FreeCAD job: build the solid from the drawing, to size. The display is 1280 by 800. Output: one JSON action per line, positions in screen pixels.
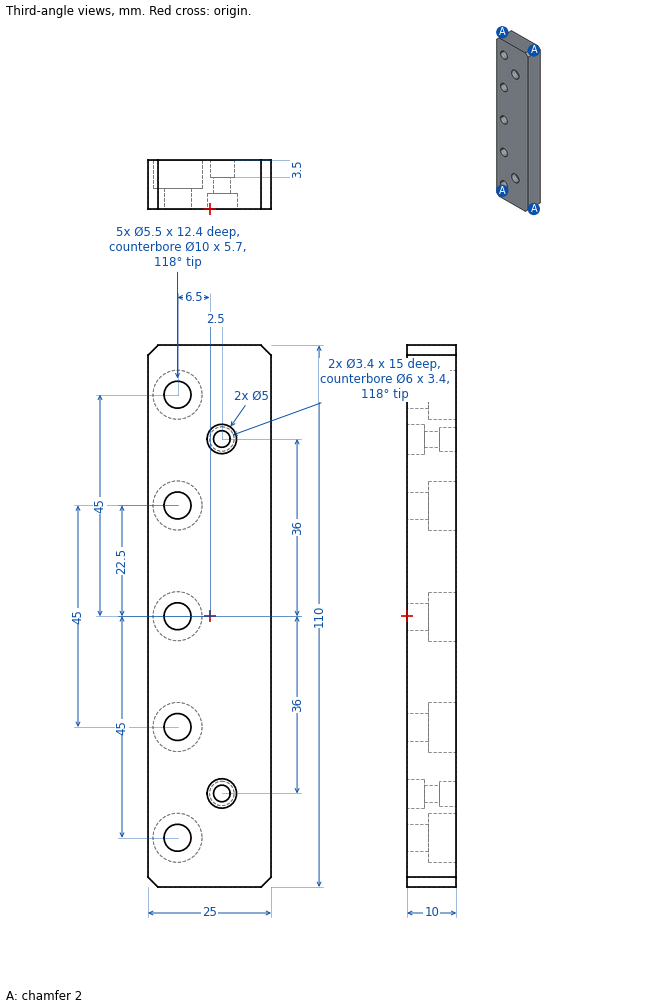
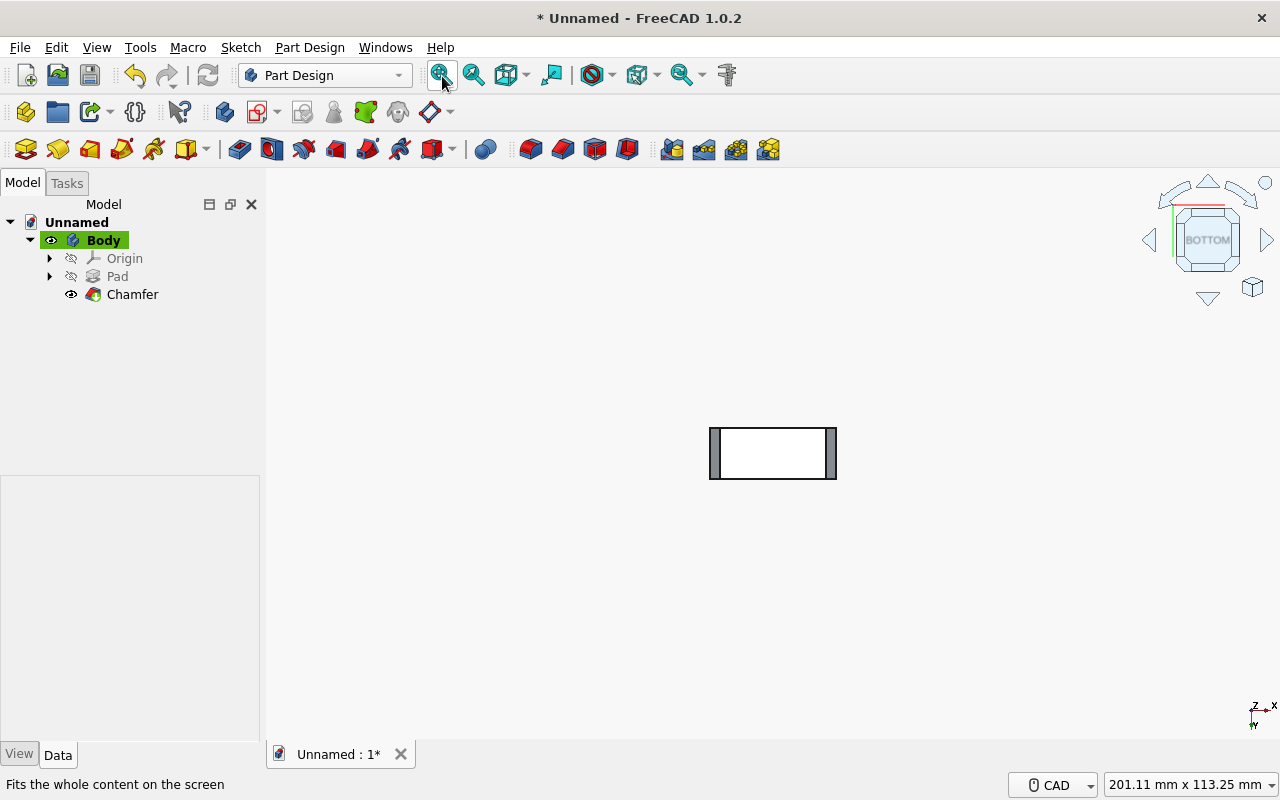
{"action": "key", "text": "4"}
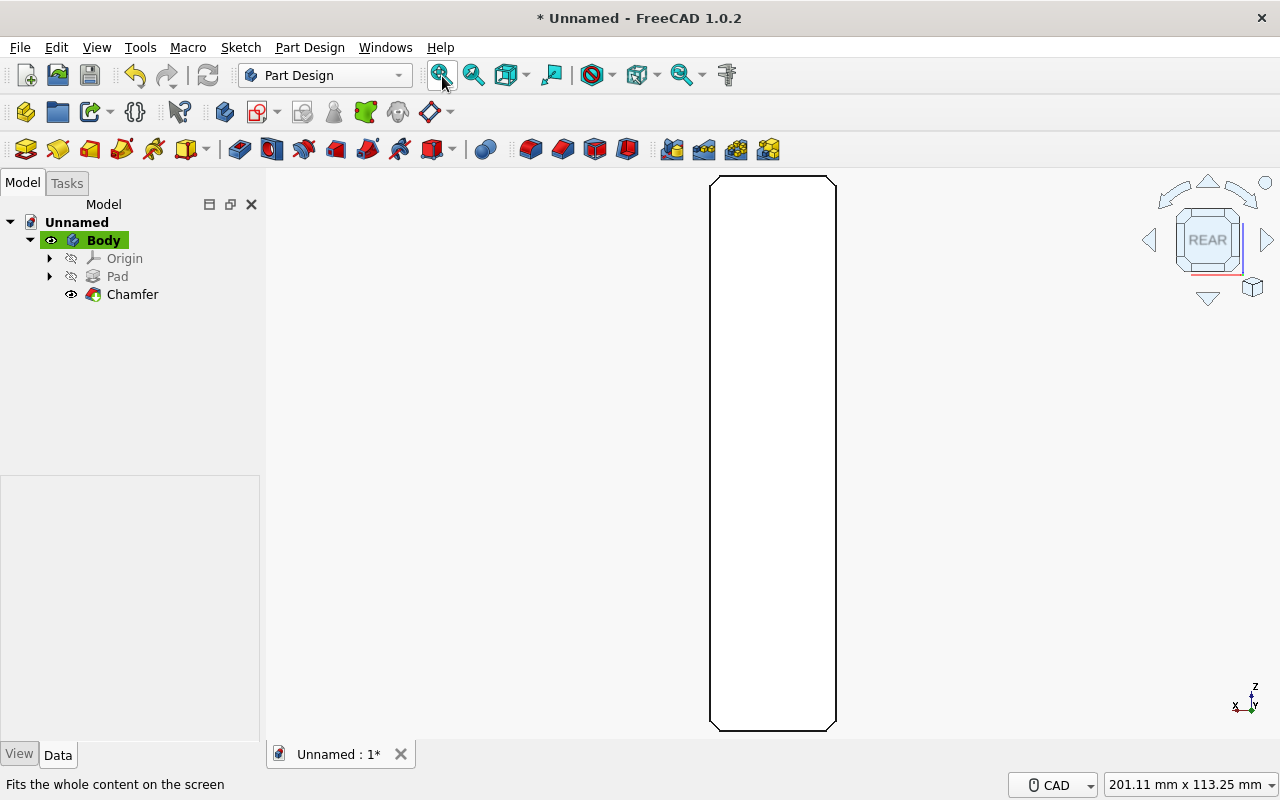
{"action": "left_click", "coordinate": [773, 294]}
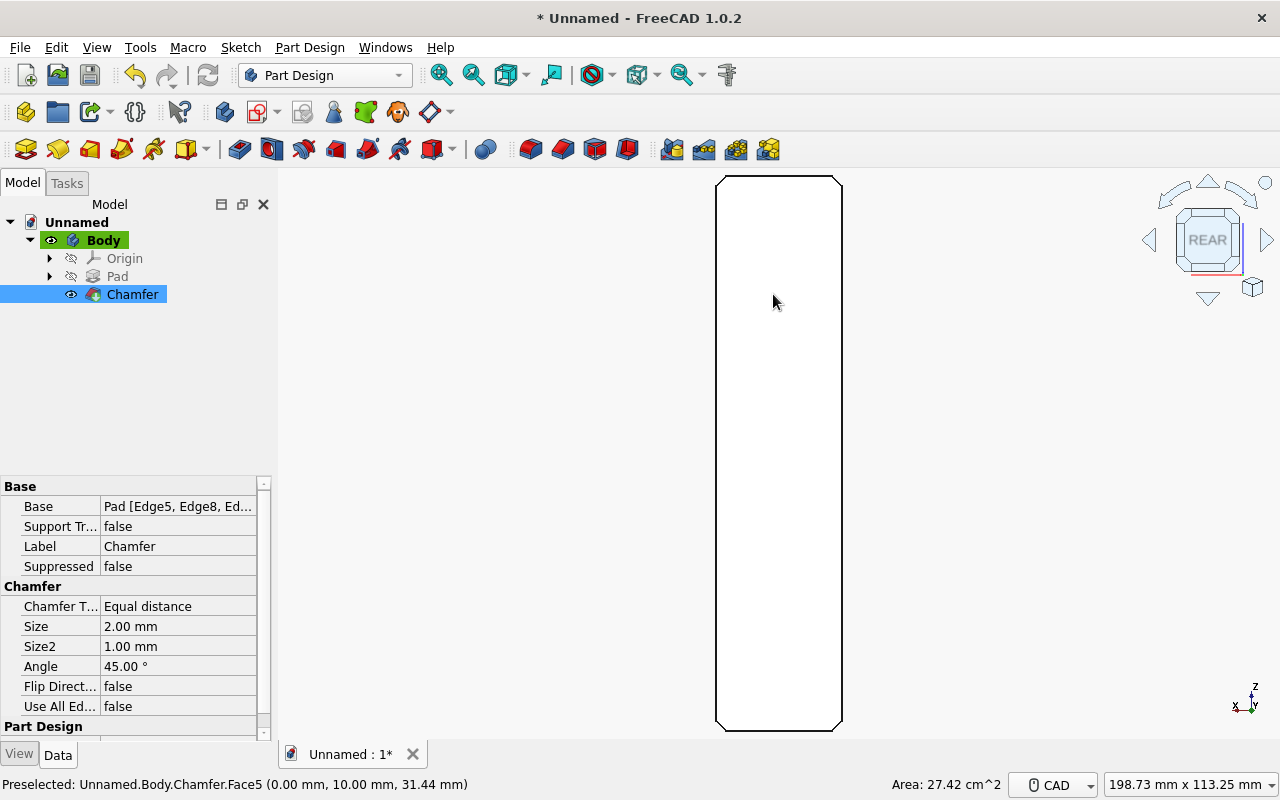
{"action": "left_click", "coordinate": [258, 112]}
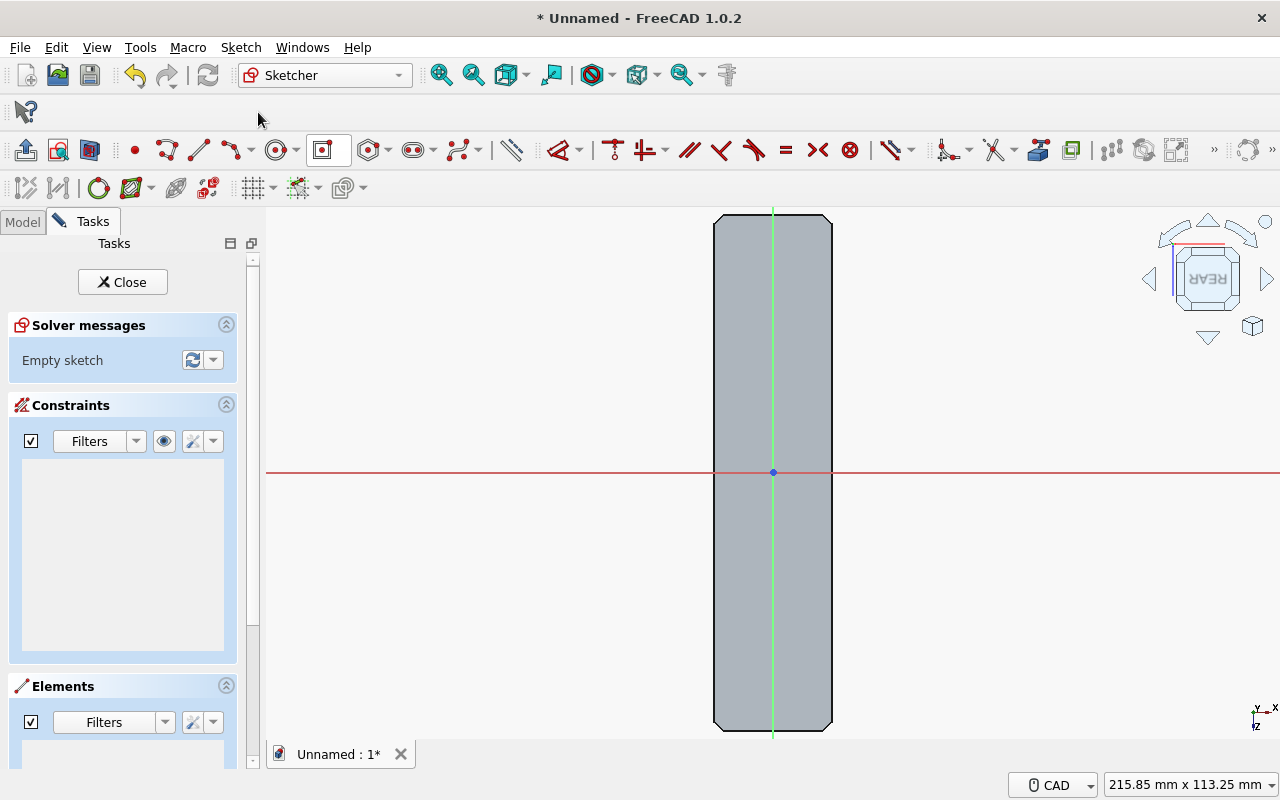
{"action": "scroll", "coordinate": [493, 473], "scroll_direction": "down", "scroll_amount": 1}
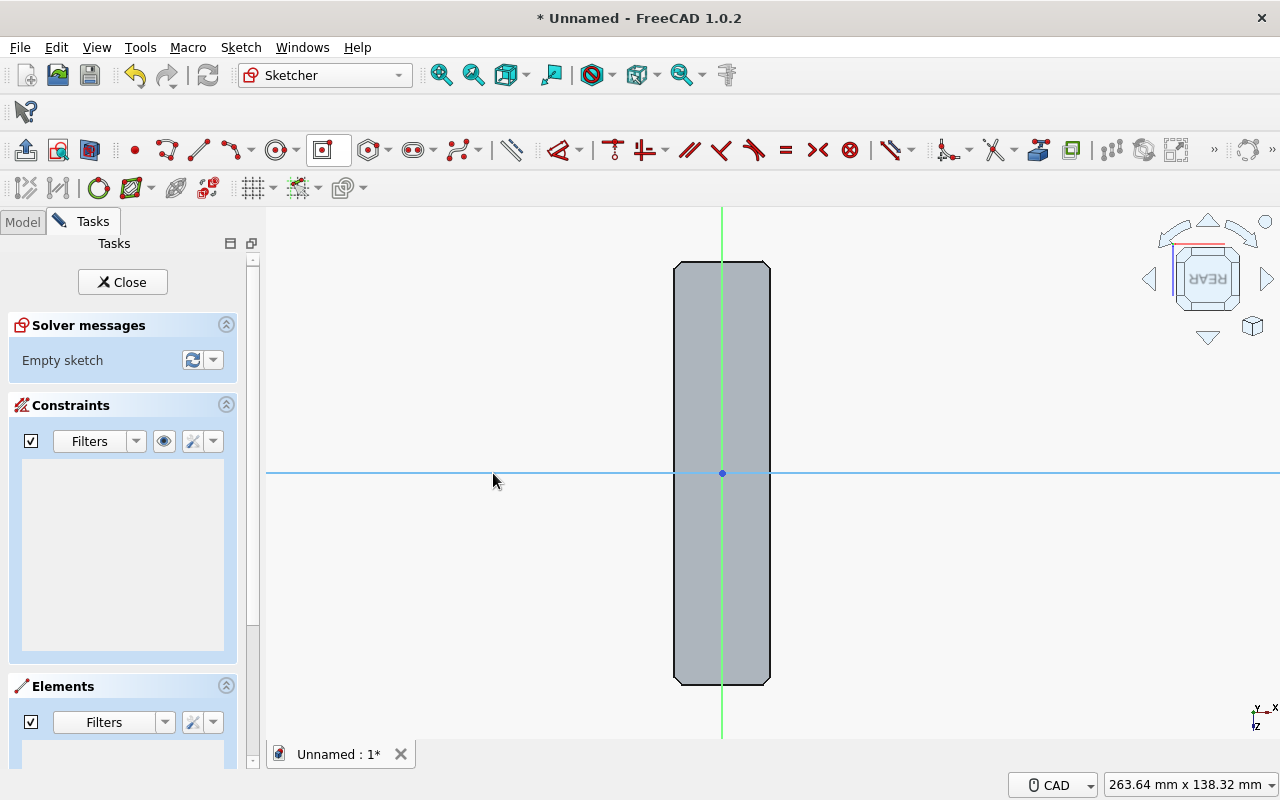
{"action": "left_click", "coordinate": [276, 150]}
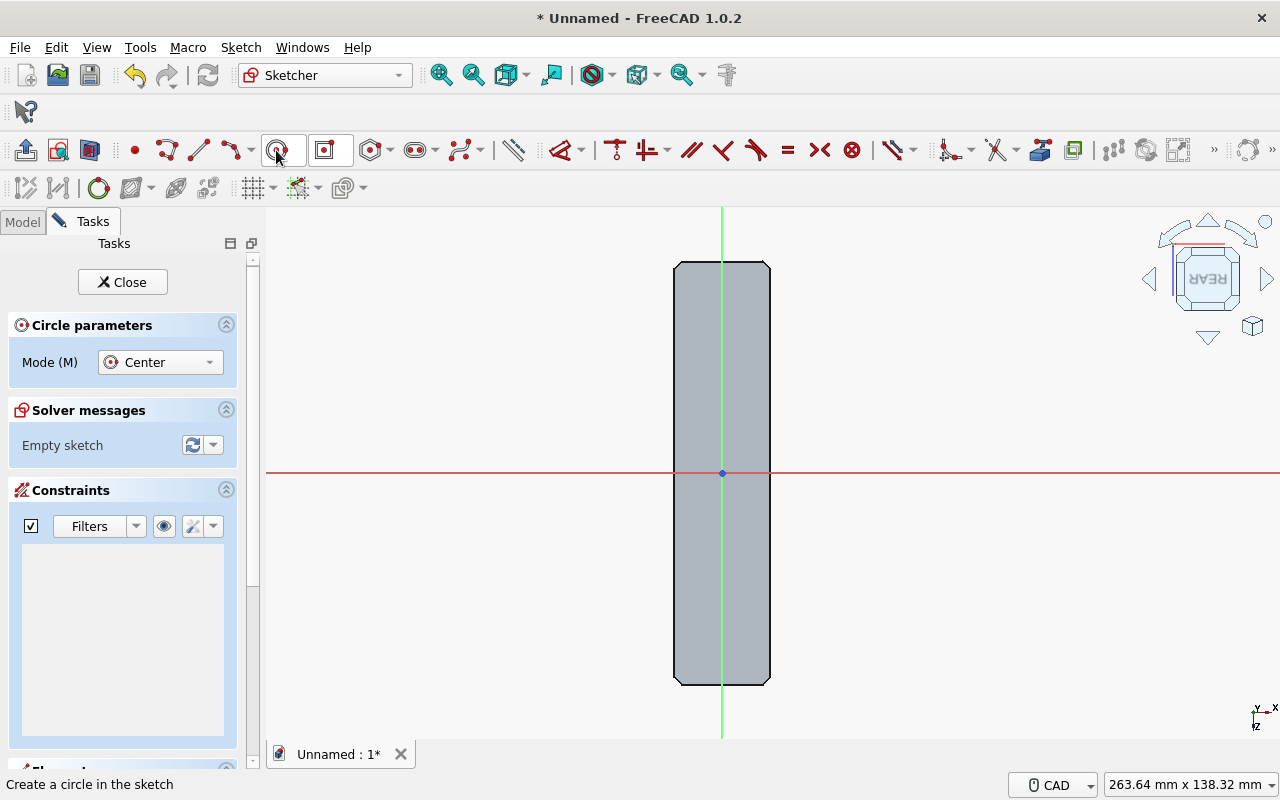
{"action": "scroll", "coordinate": [697, 646], "scroll_direction": "up", "scroll_amount": 4}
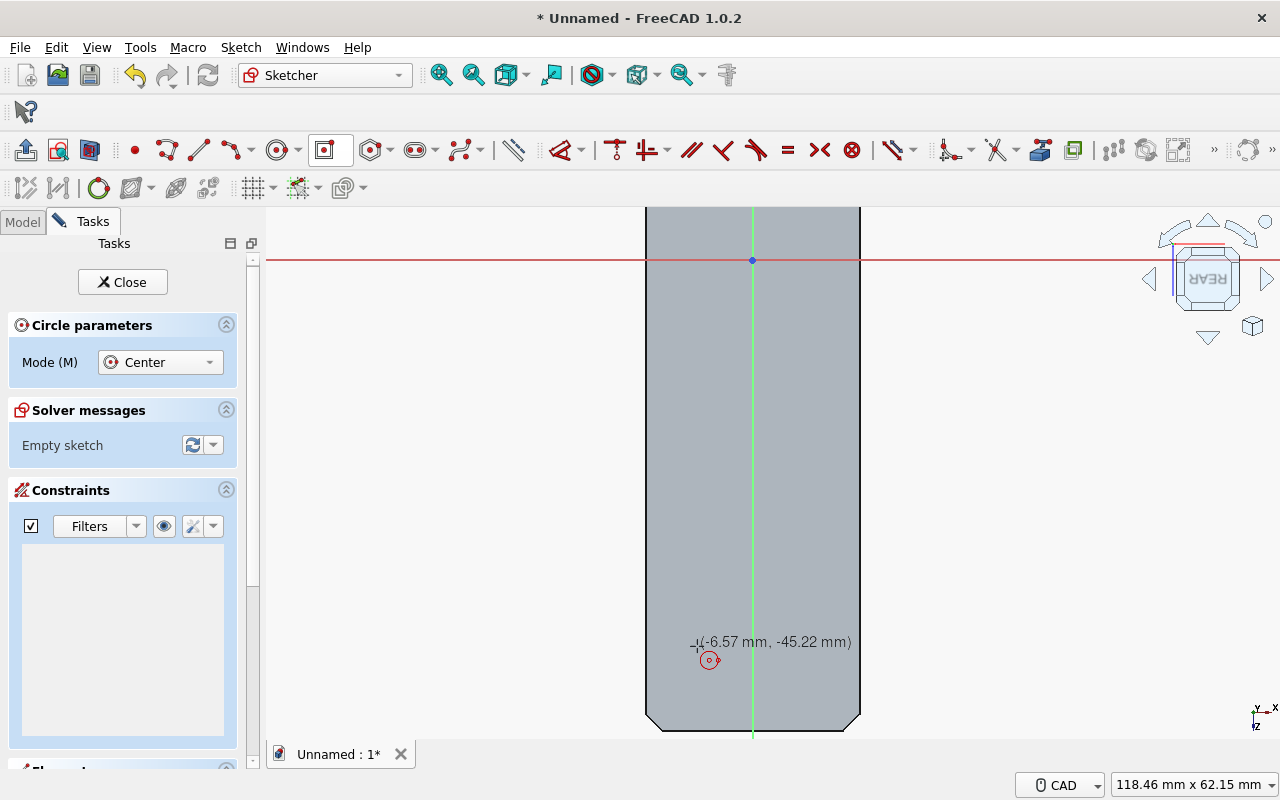
{"action": "left_click", "coordinate": [697, 645]}
{"action": "mouse_move", "coordinate": [714, 629]}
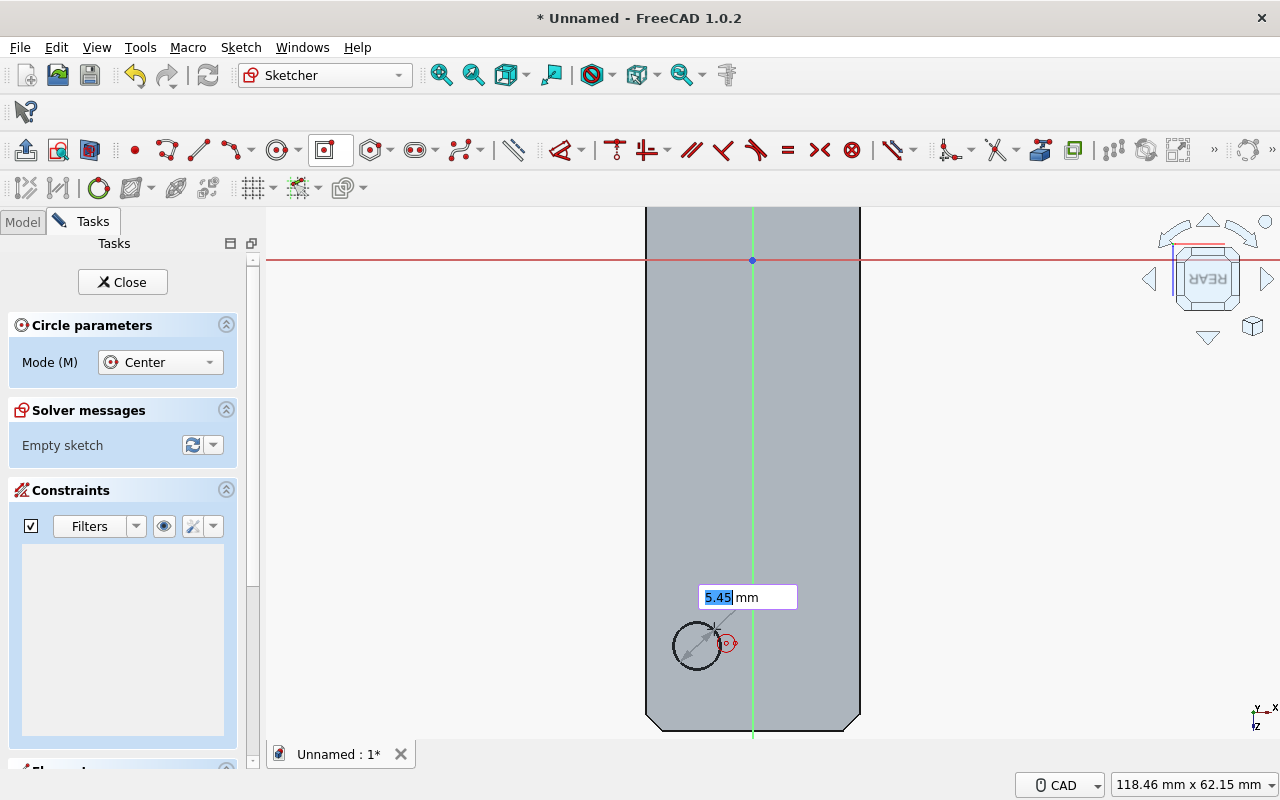
{"action": "type", "text": "5.5"}
{"action": "key", "text": "Return"}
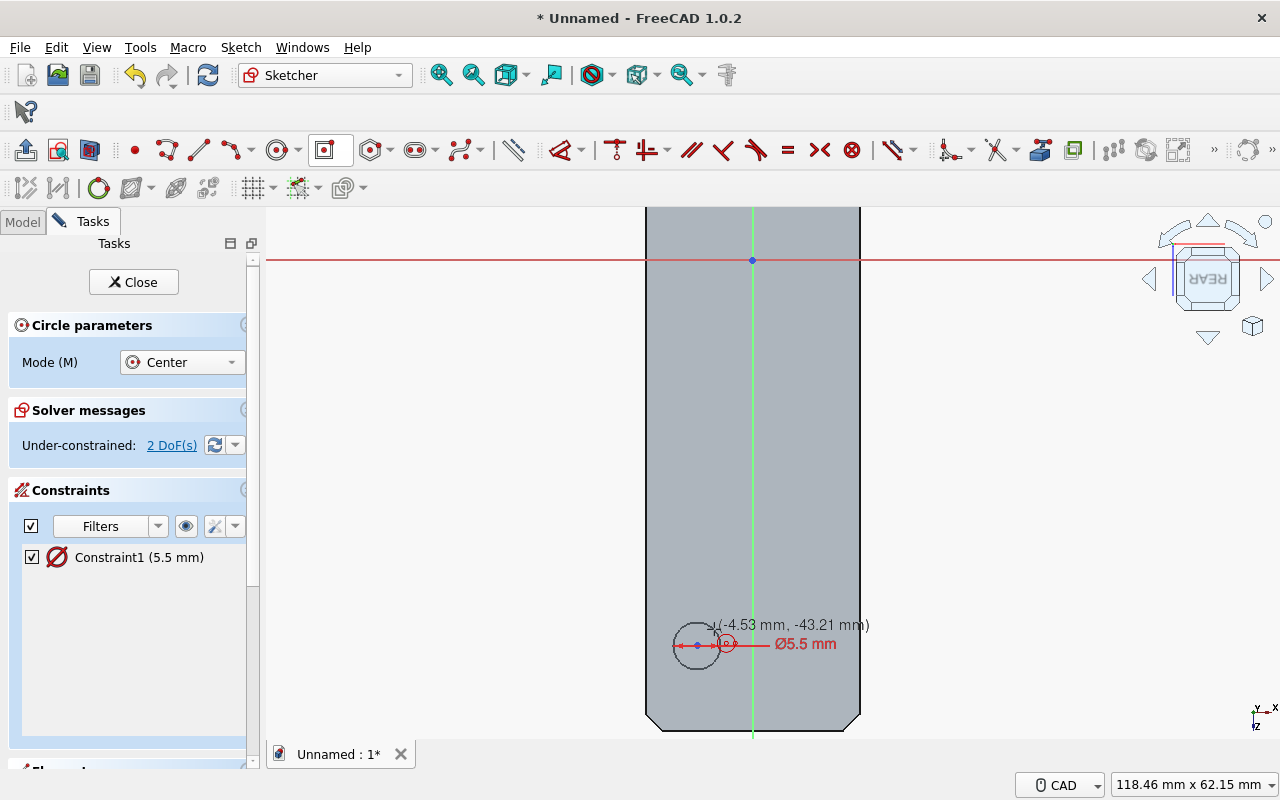
{"action": "left_click", "coordinate": [697, 260]}
{"action": "mouse_move", "coordinate": [714, 244]}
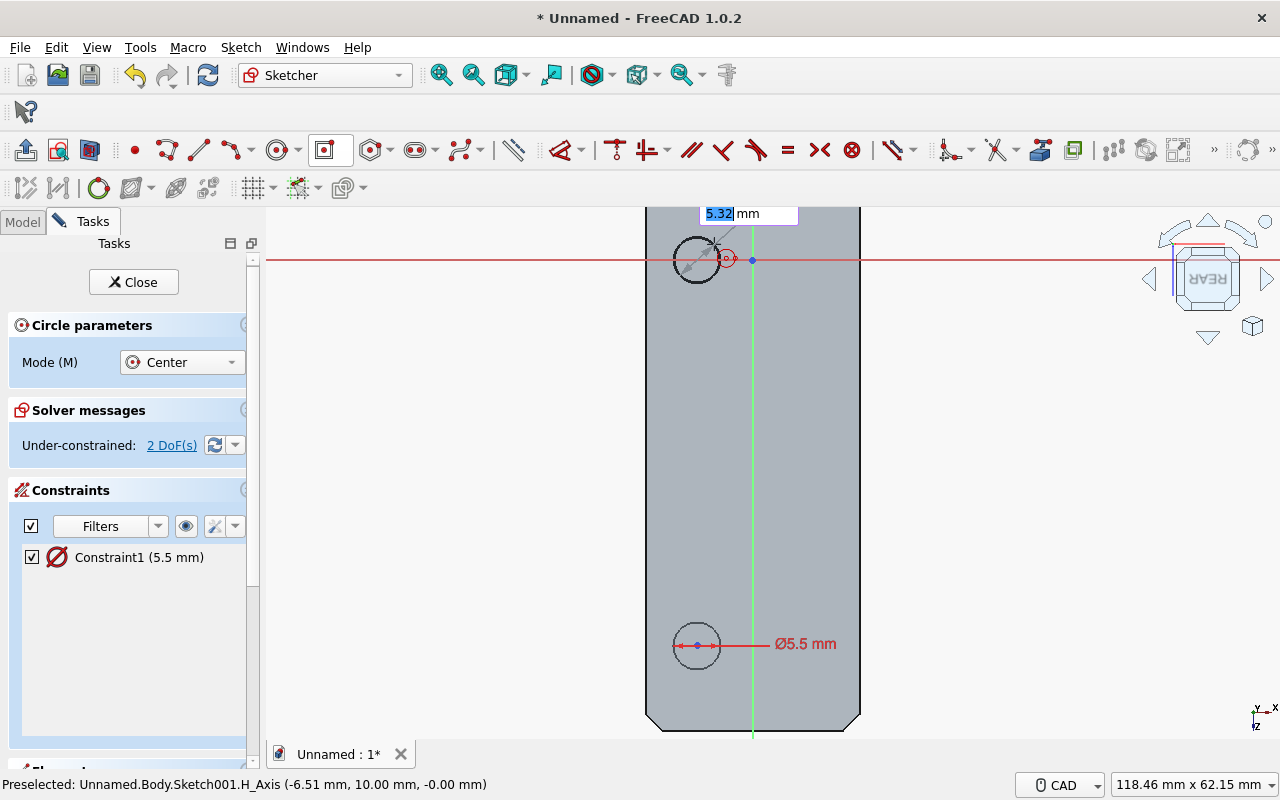
{"action": "type", "text": "5.5"}
{"action": "key", "text": "Return"}